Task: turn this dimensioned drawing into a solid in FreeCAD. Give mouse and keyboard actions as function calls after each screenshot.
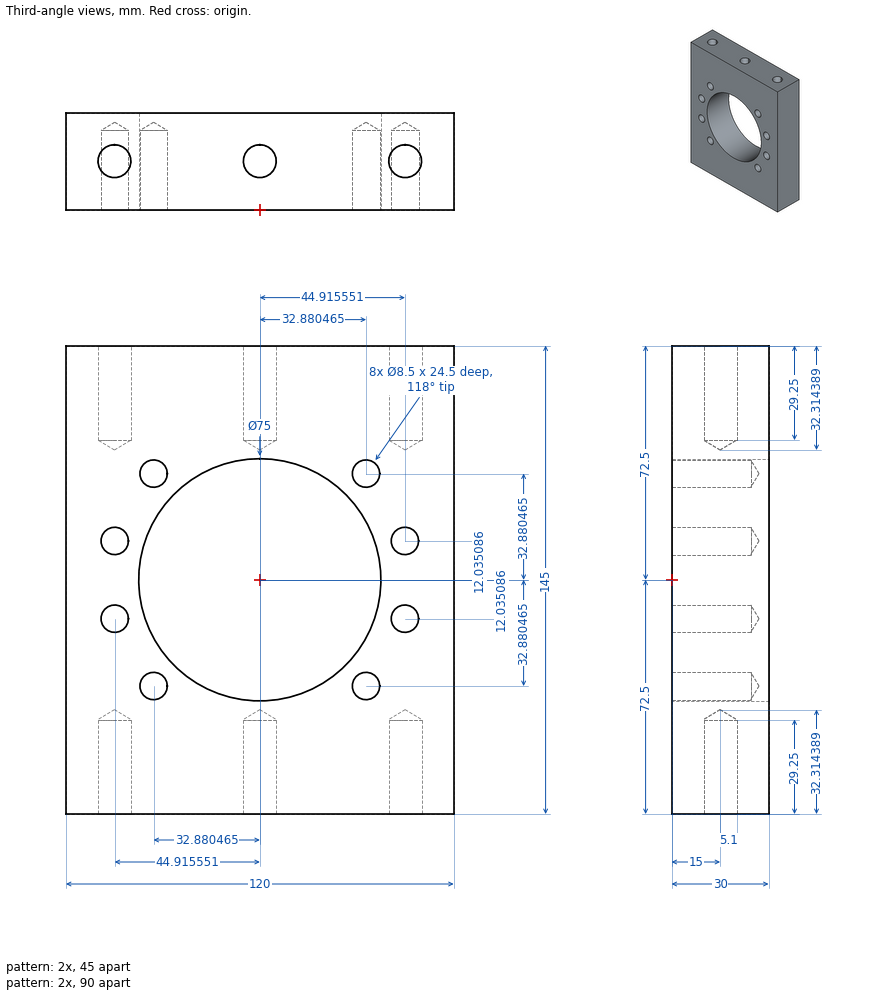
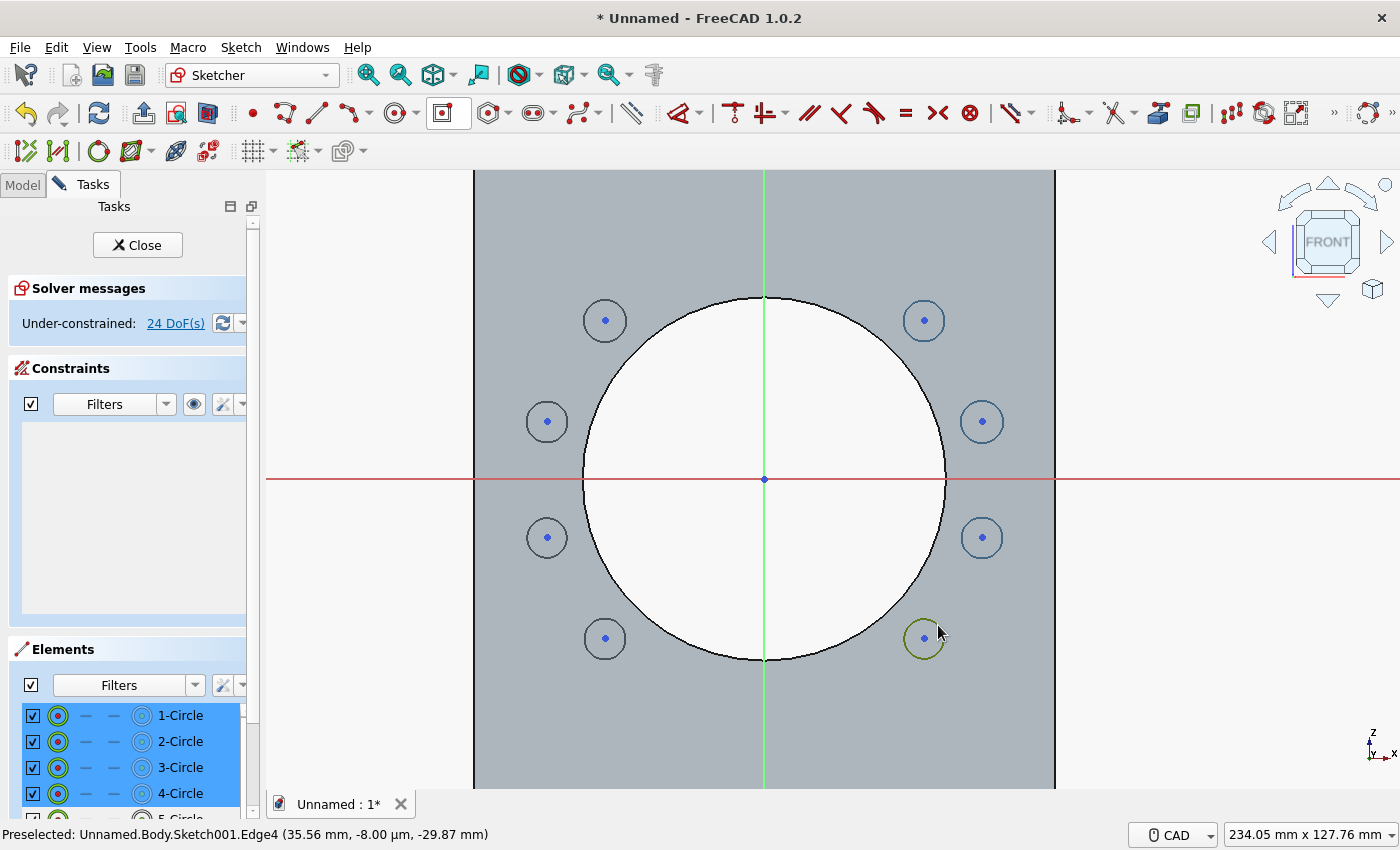
click(619, 624)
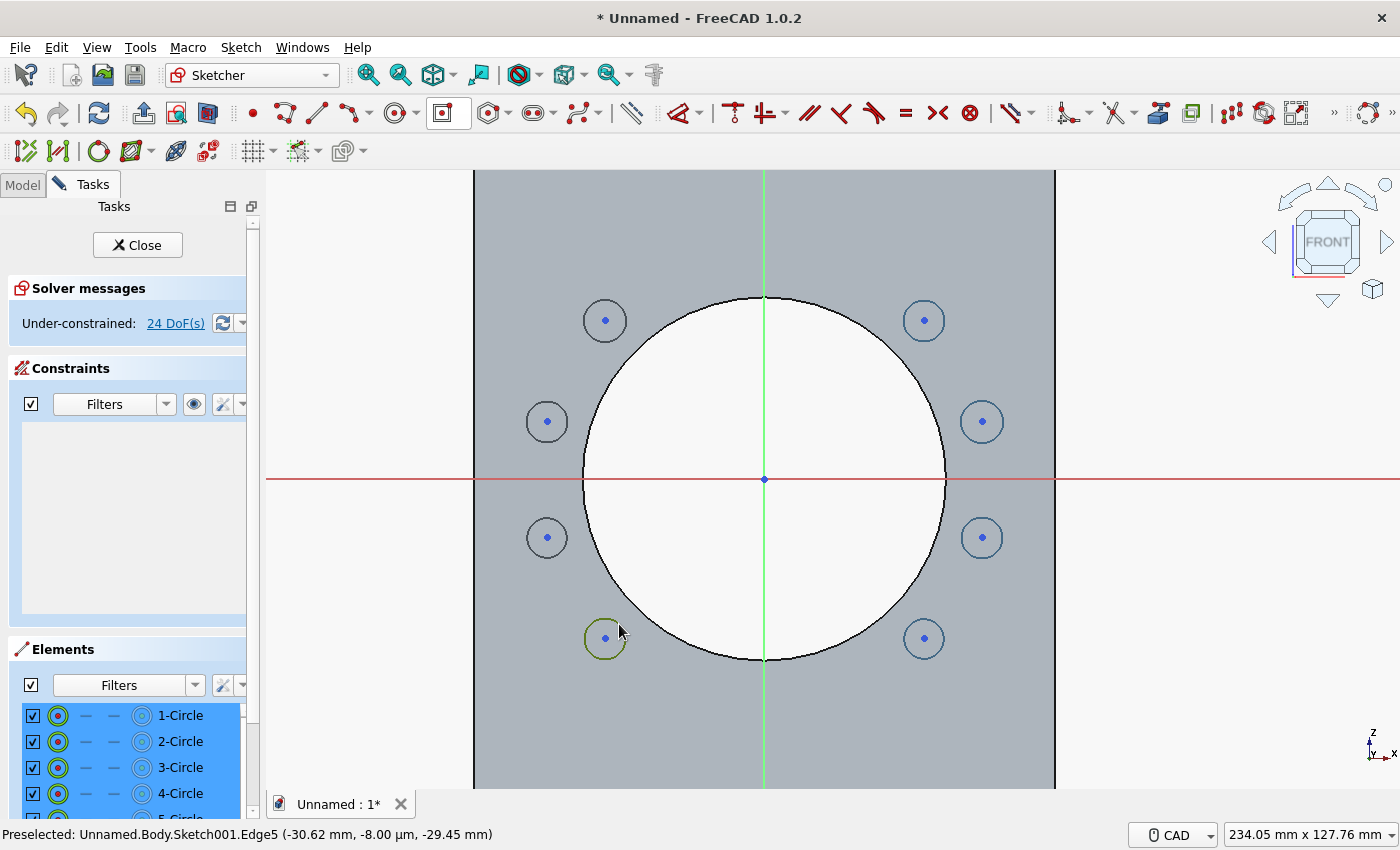
click(561, 524)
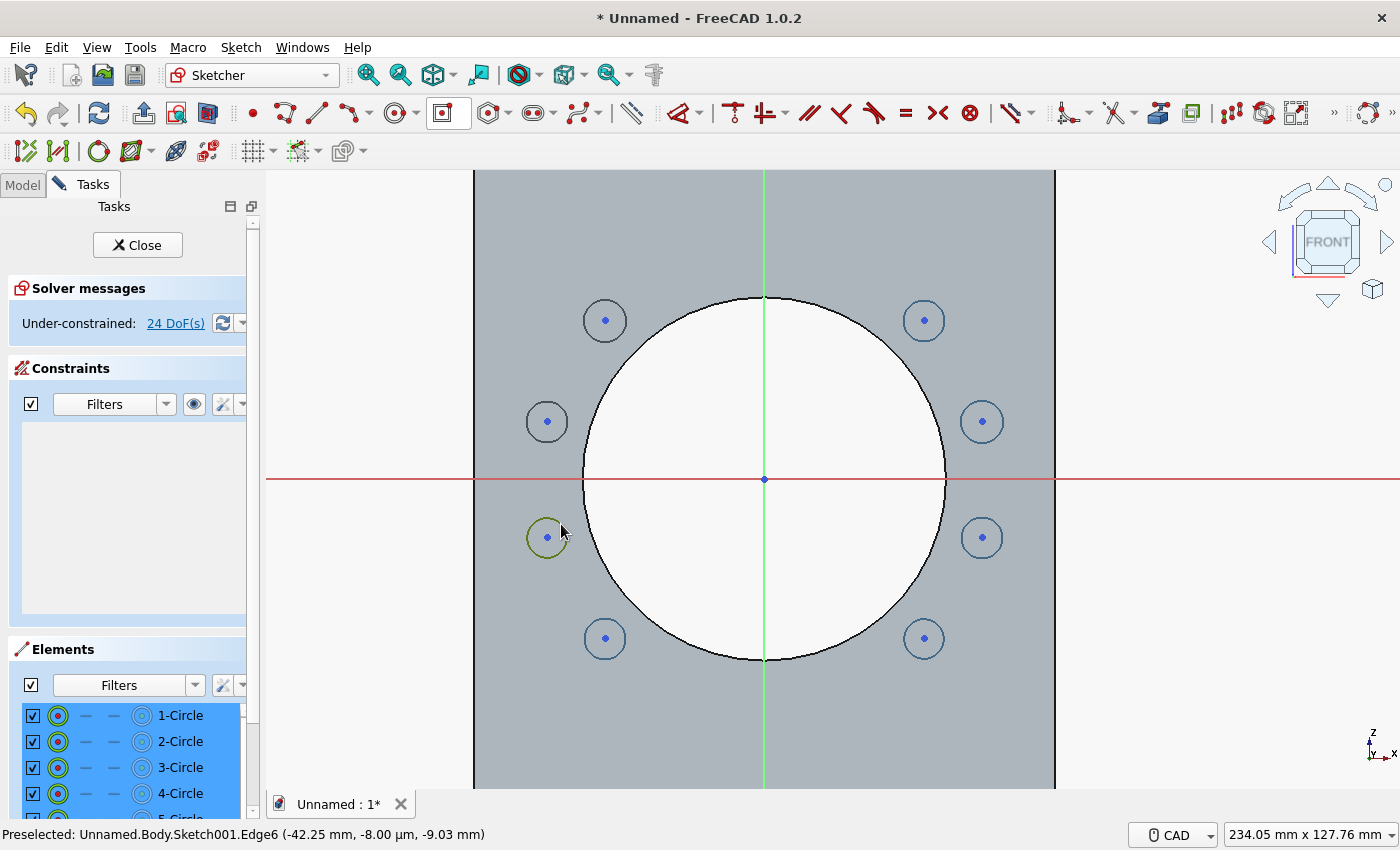
click(561, 407)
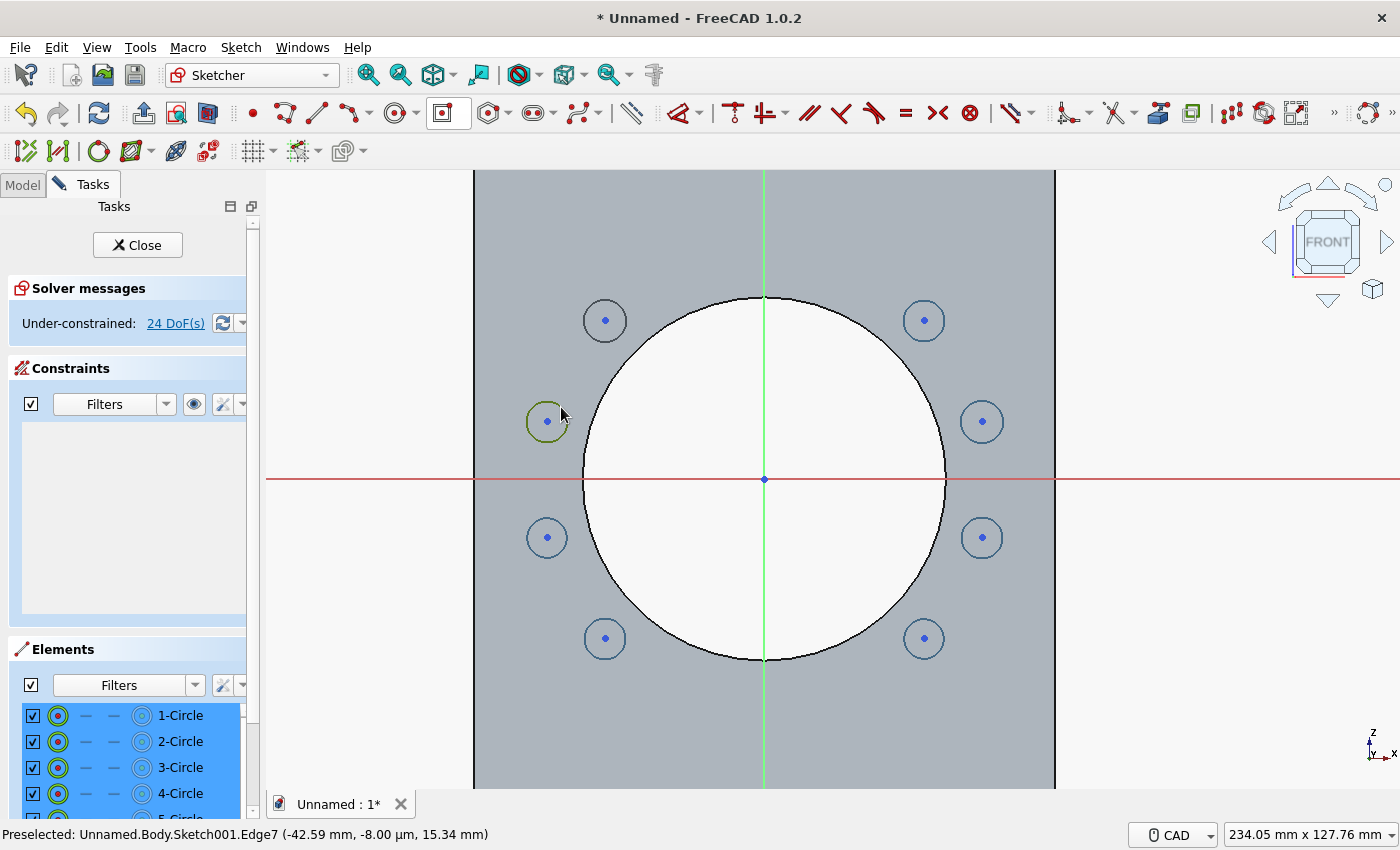
click(620, 306)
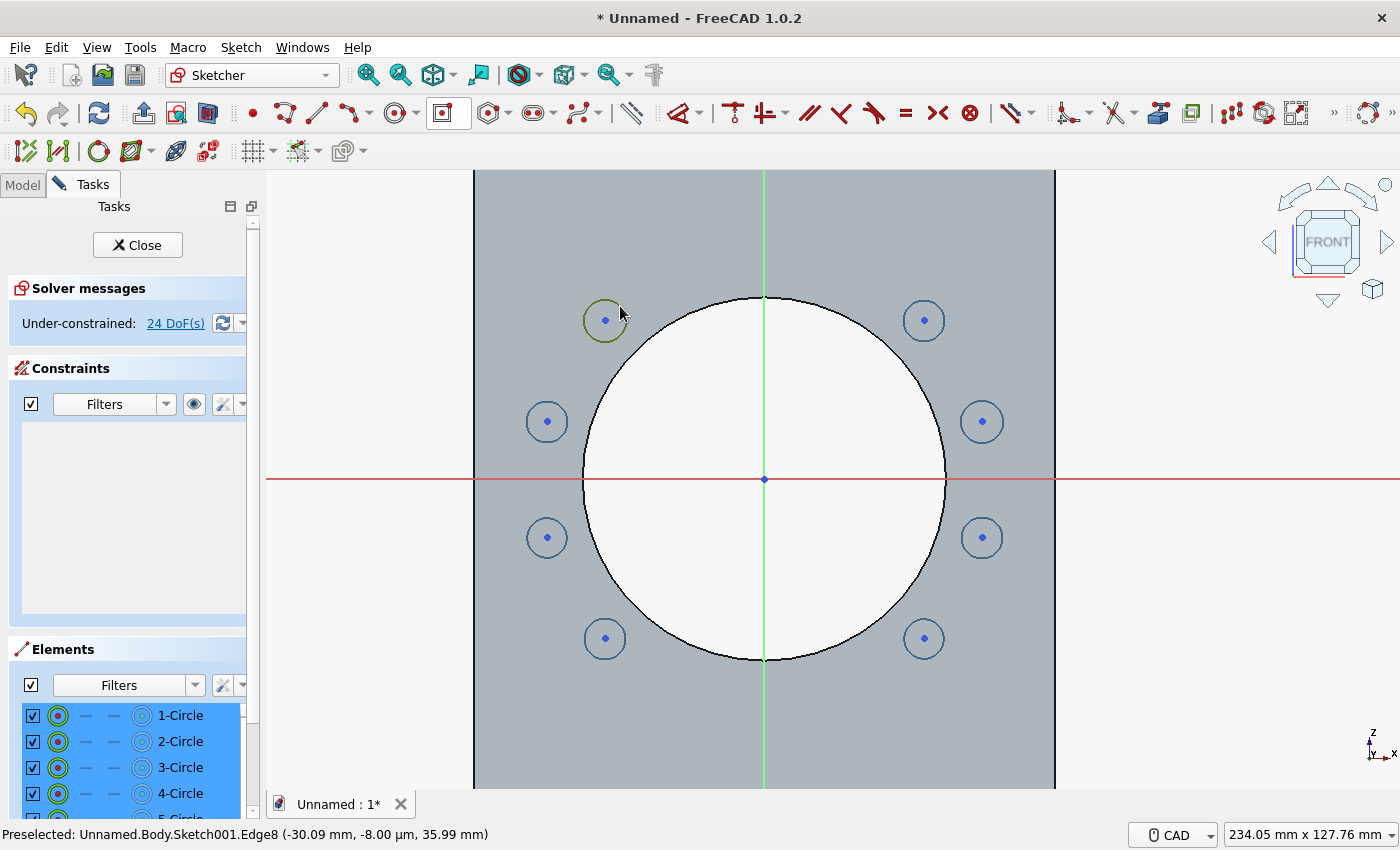
click(906, 114)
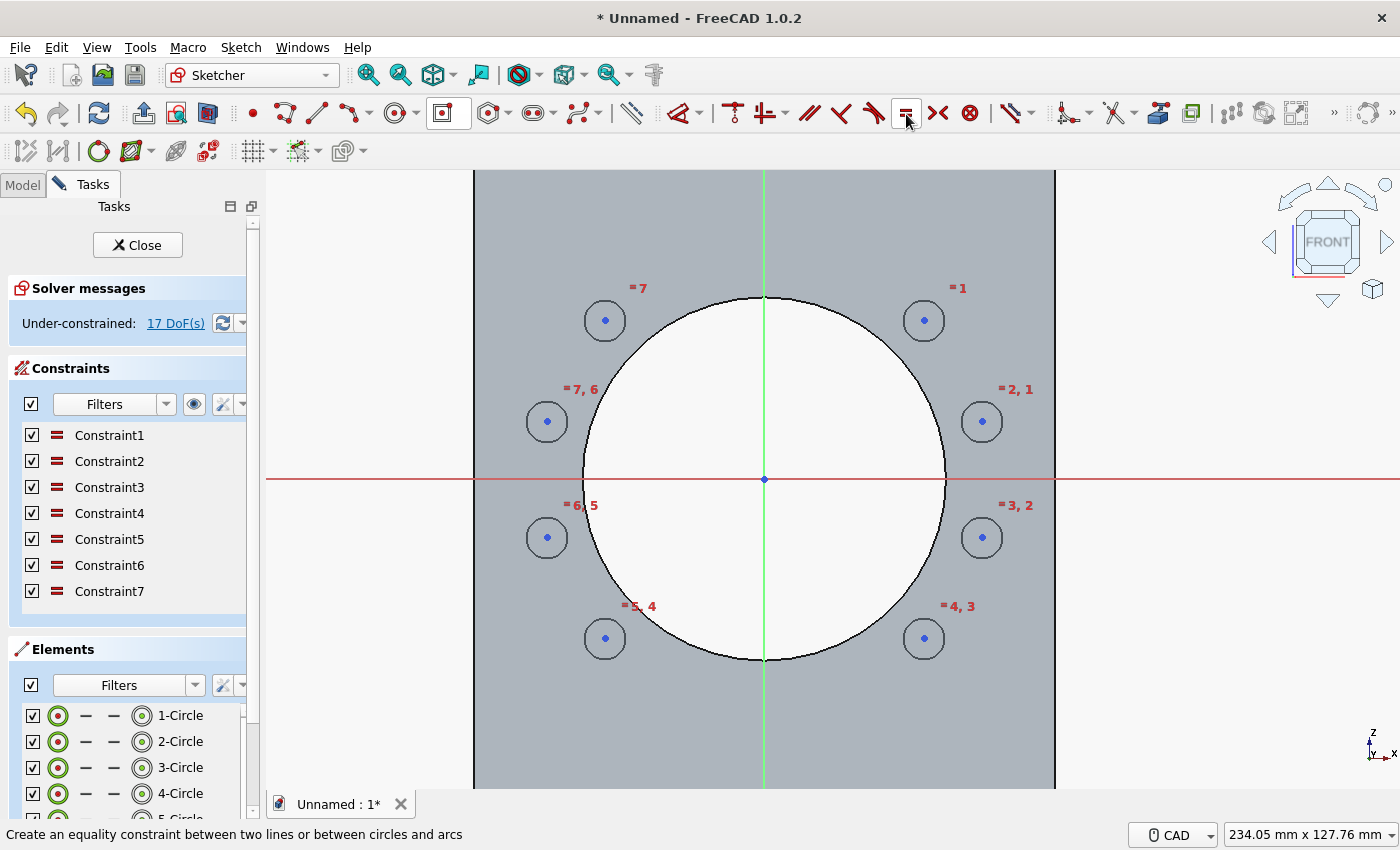
click(982, 422)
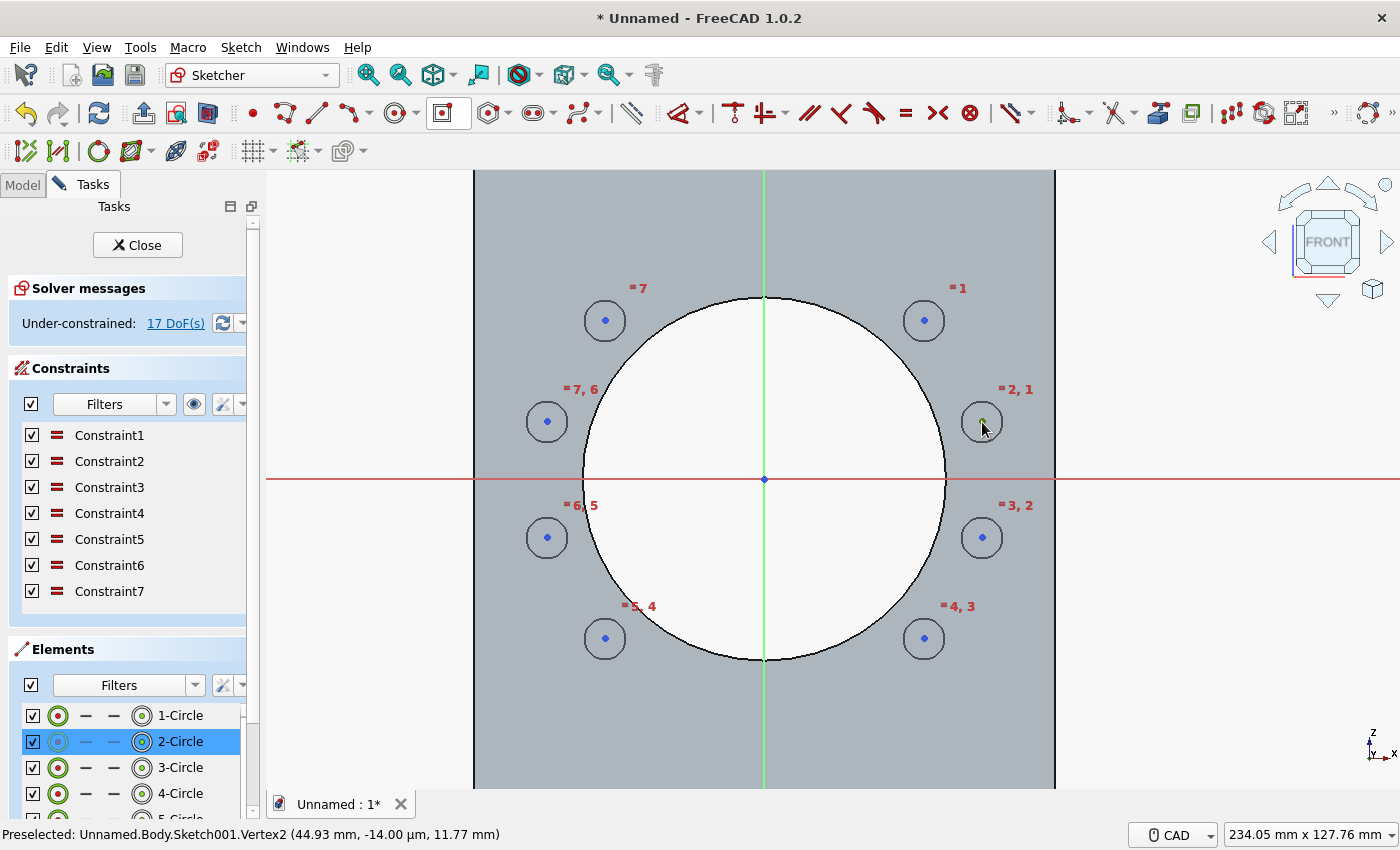
click(982, 538)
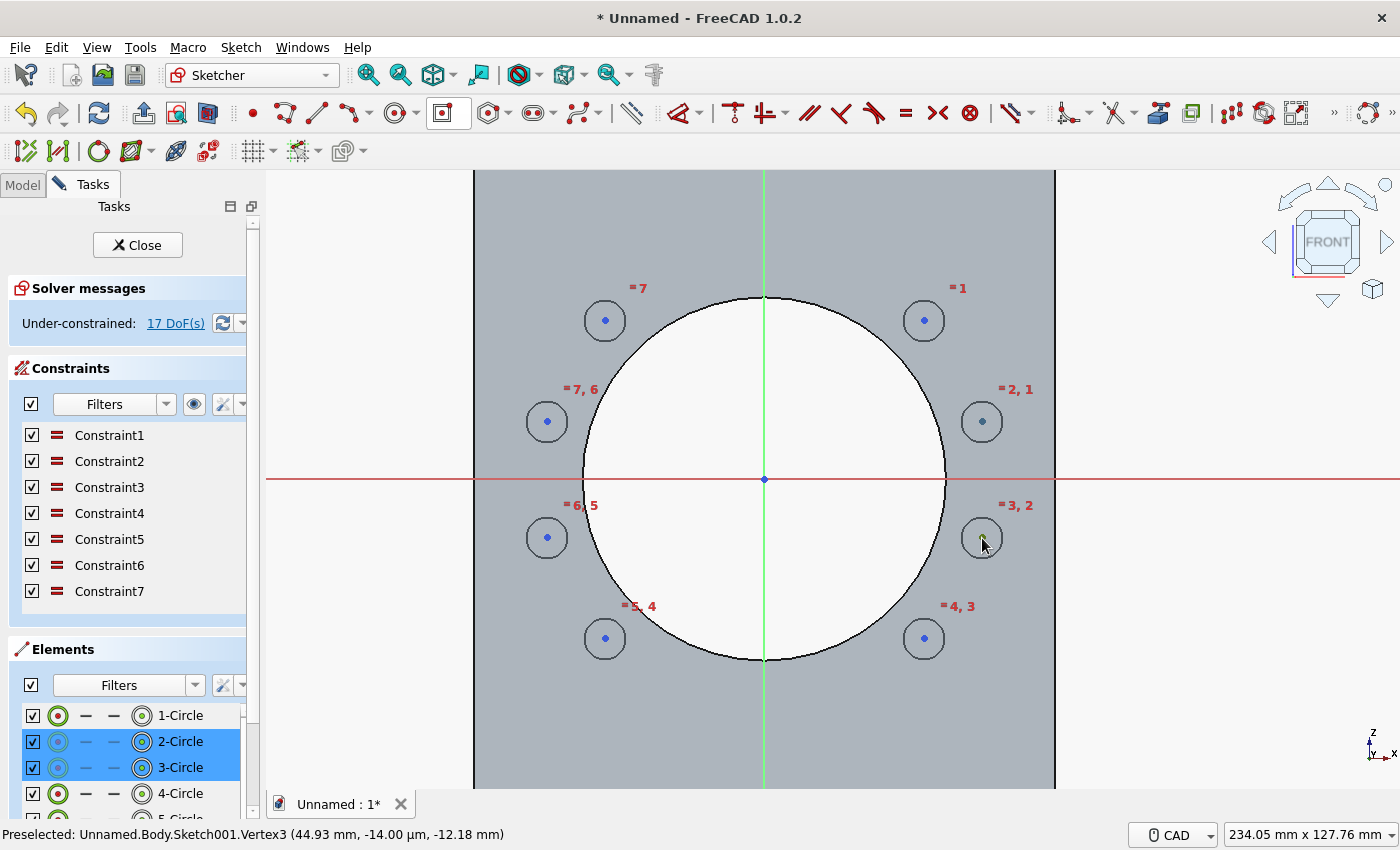
click(788, 114)